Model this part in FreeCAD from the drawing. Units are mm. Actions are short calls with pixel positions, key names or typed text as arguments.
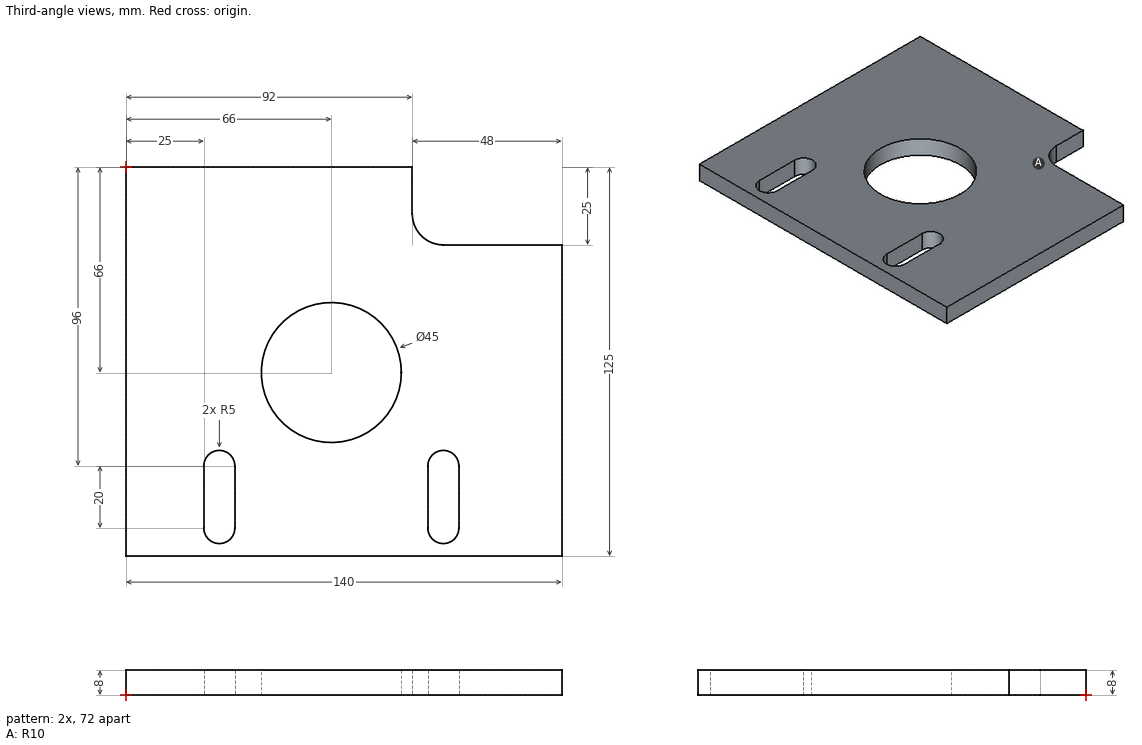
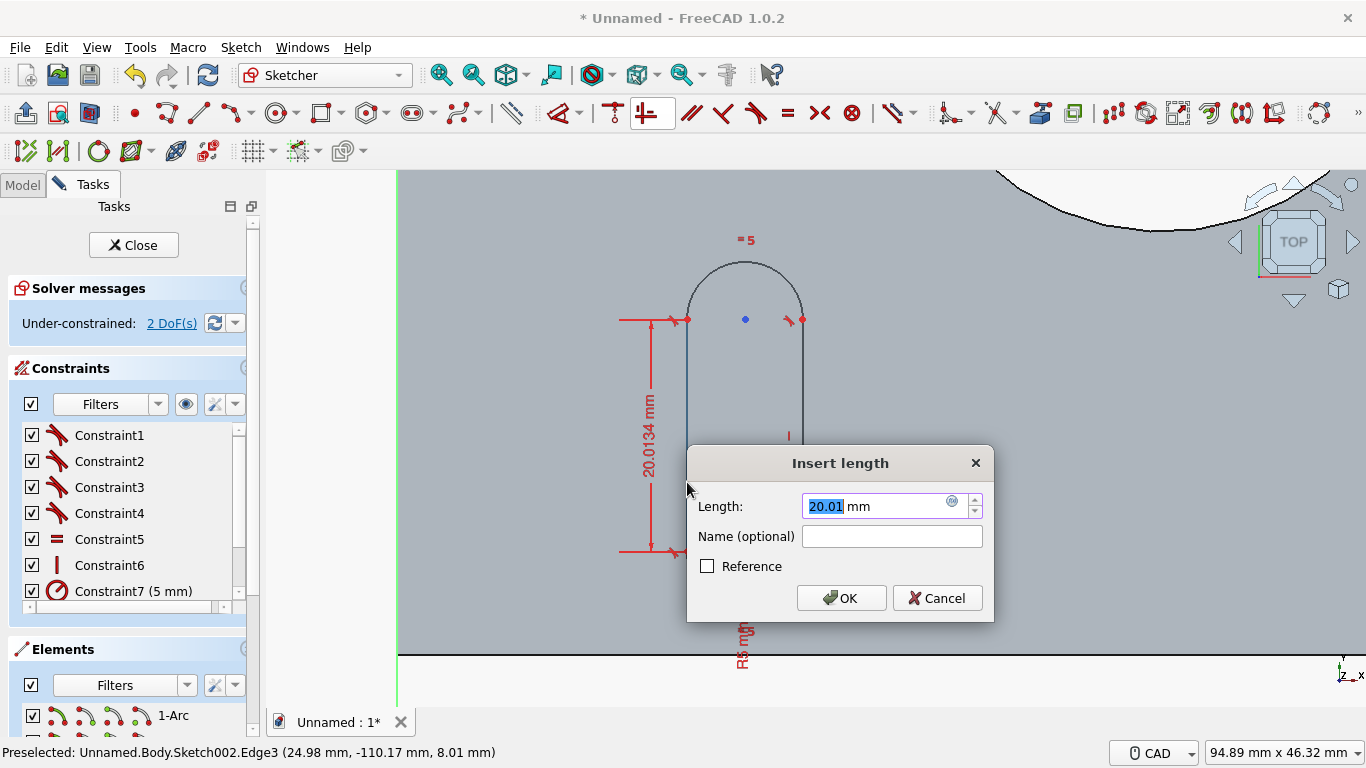
text(20)
key(Return)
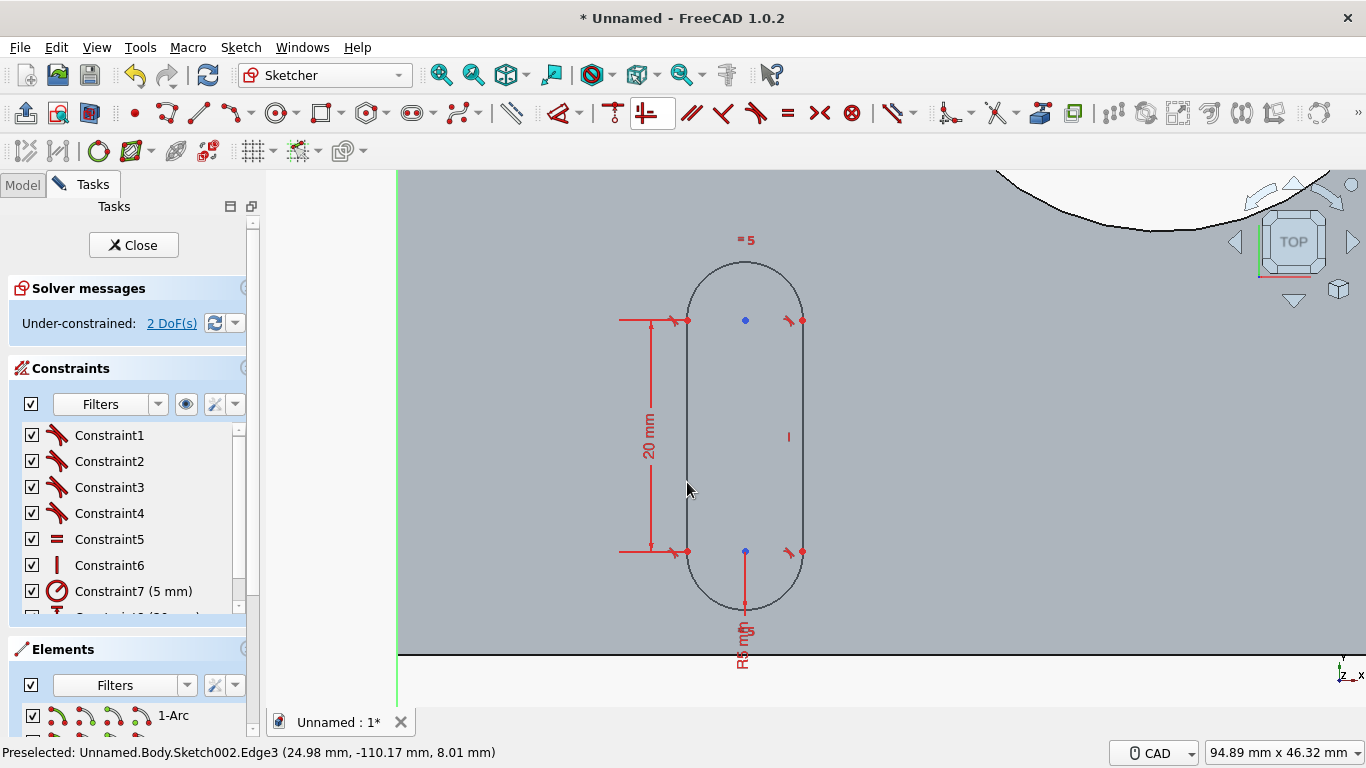
click(687, 552)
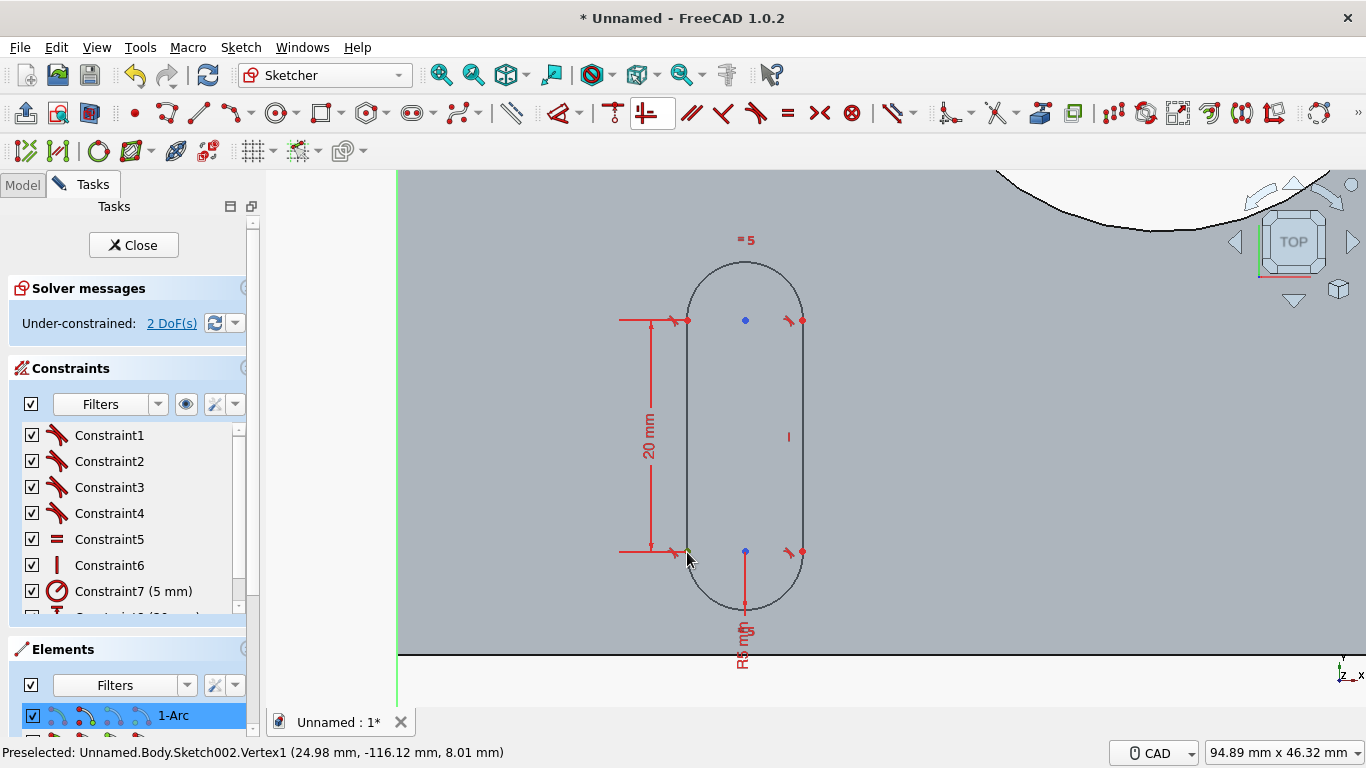
key(l)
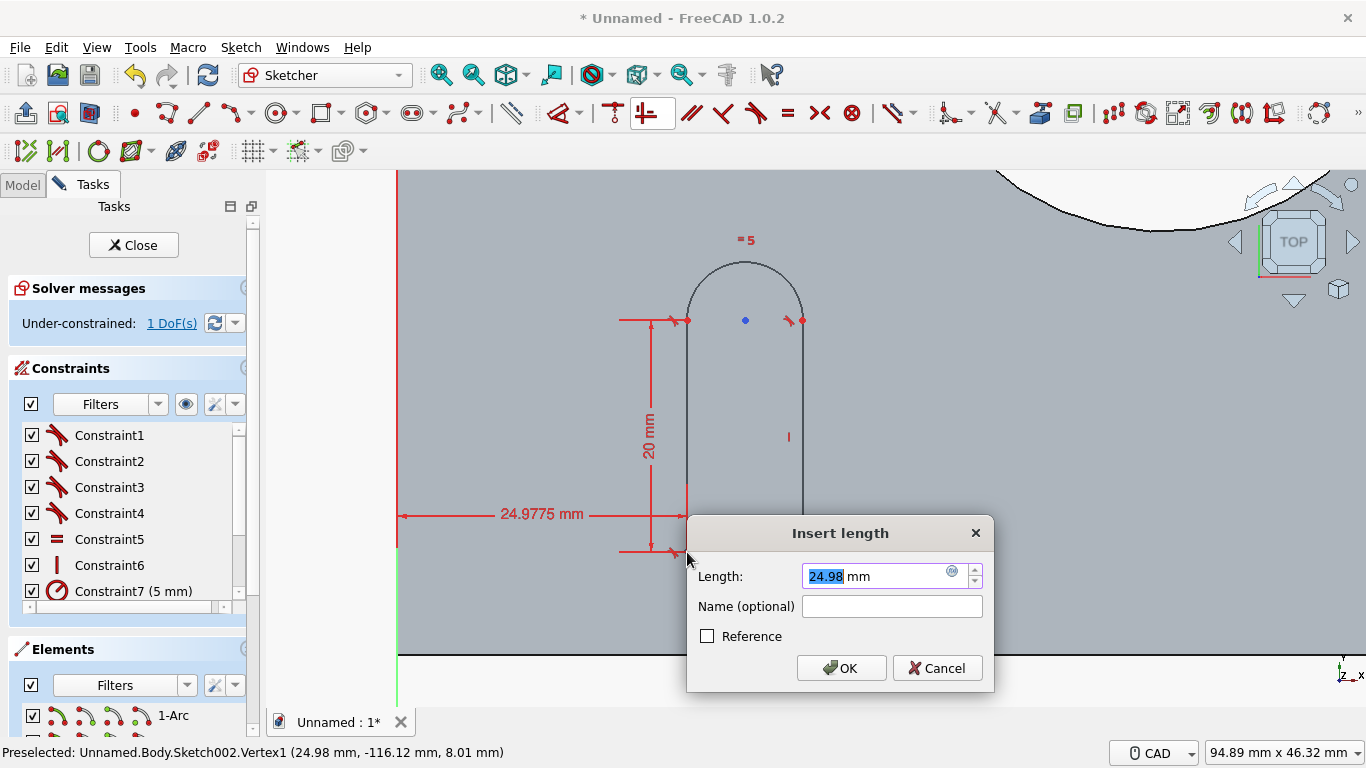
text(25)
key(Return)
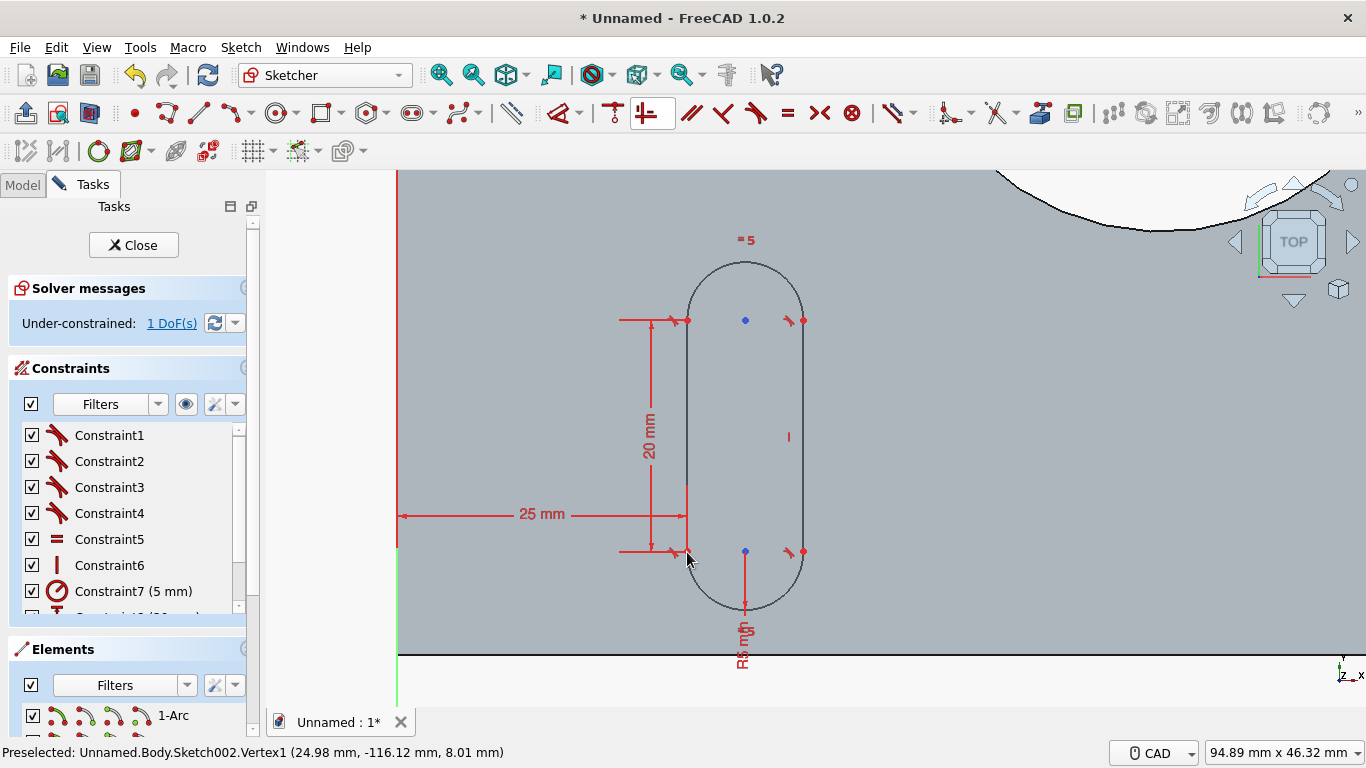
click(803, 320)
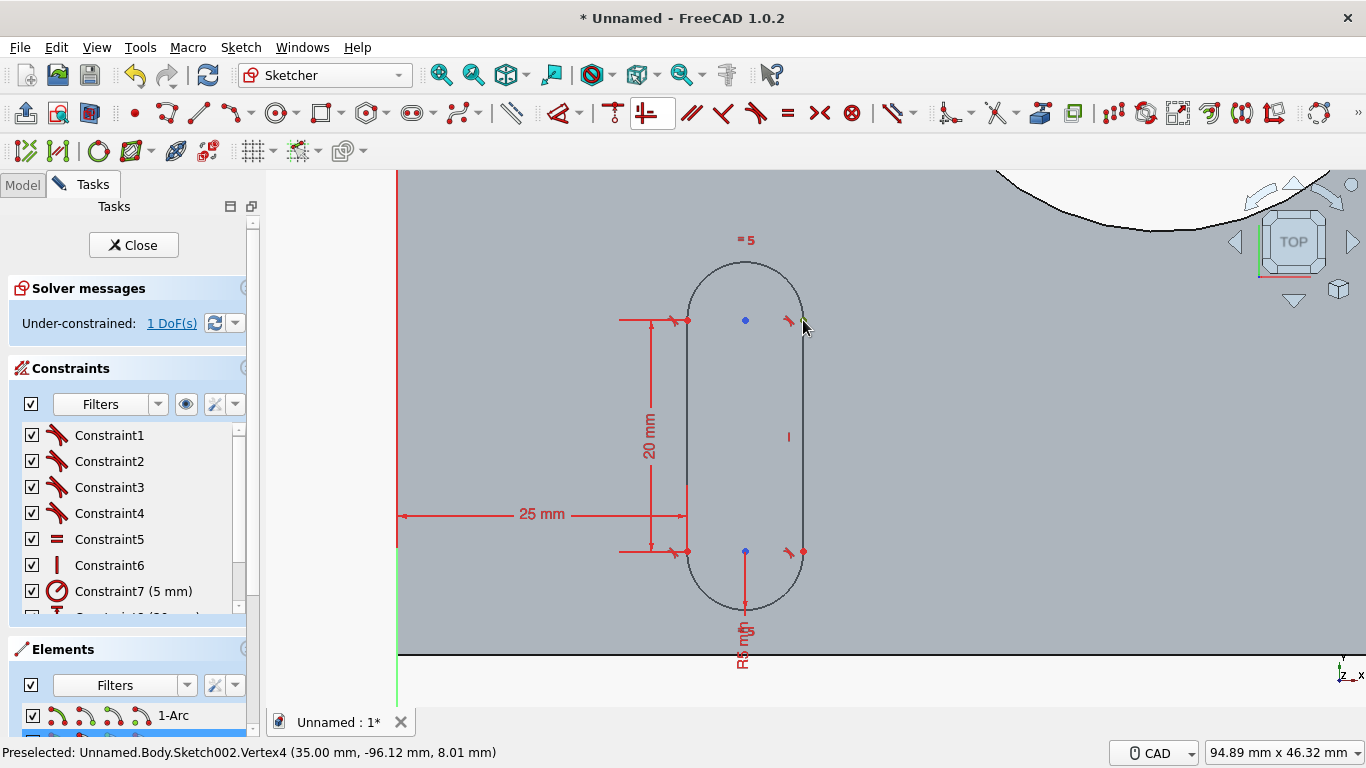
click(582, 114)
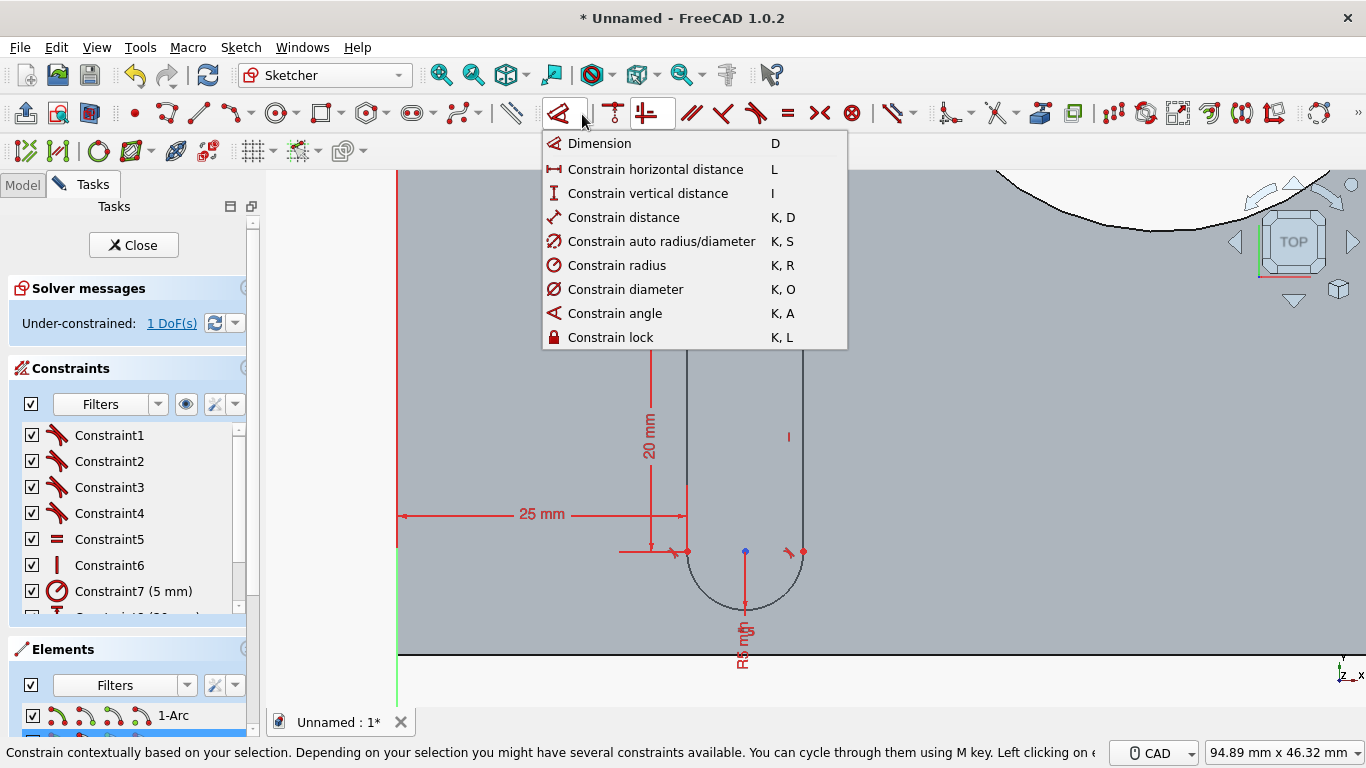
click(695, 193)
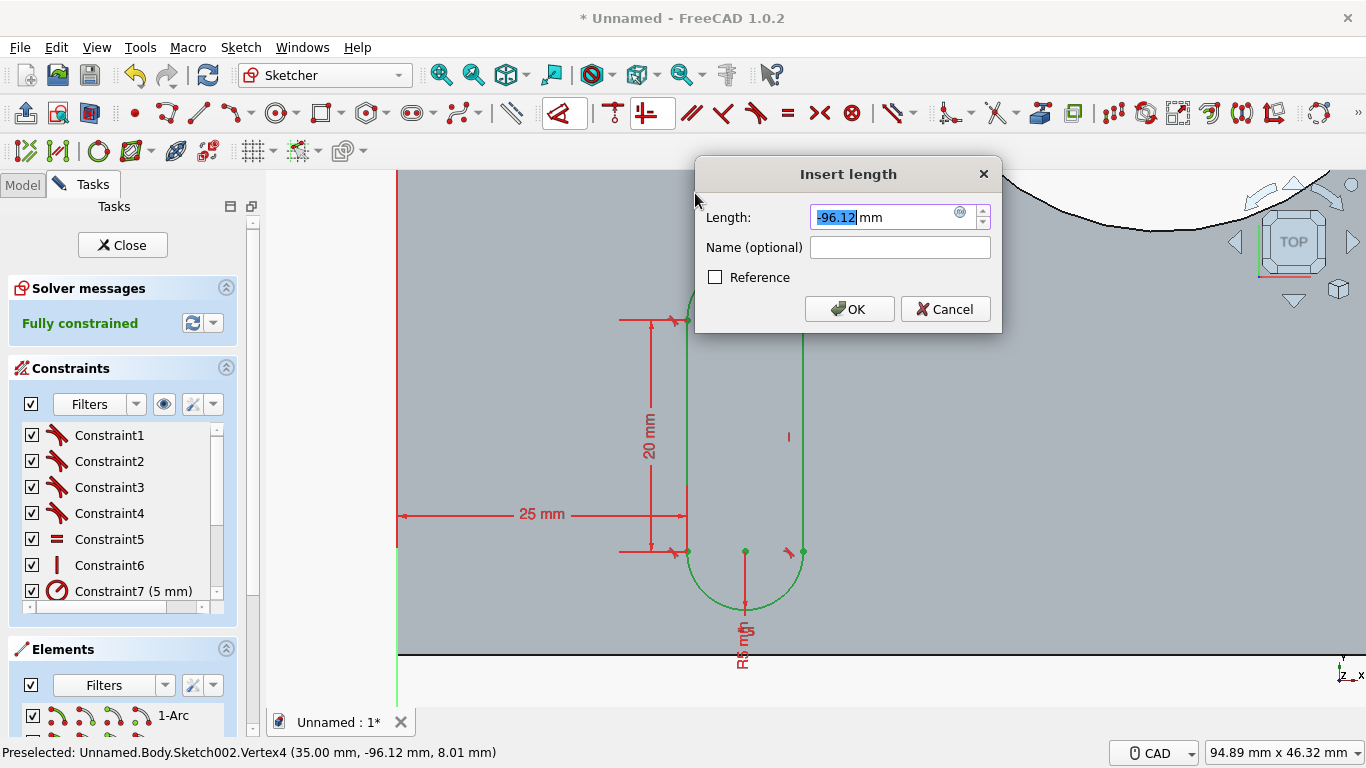
text(-96)
key(Return)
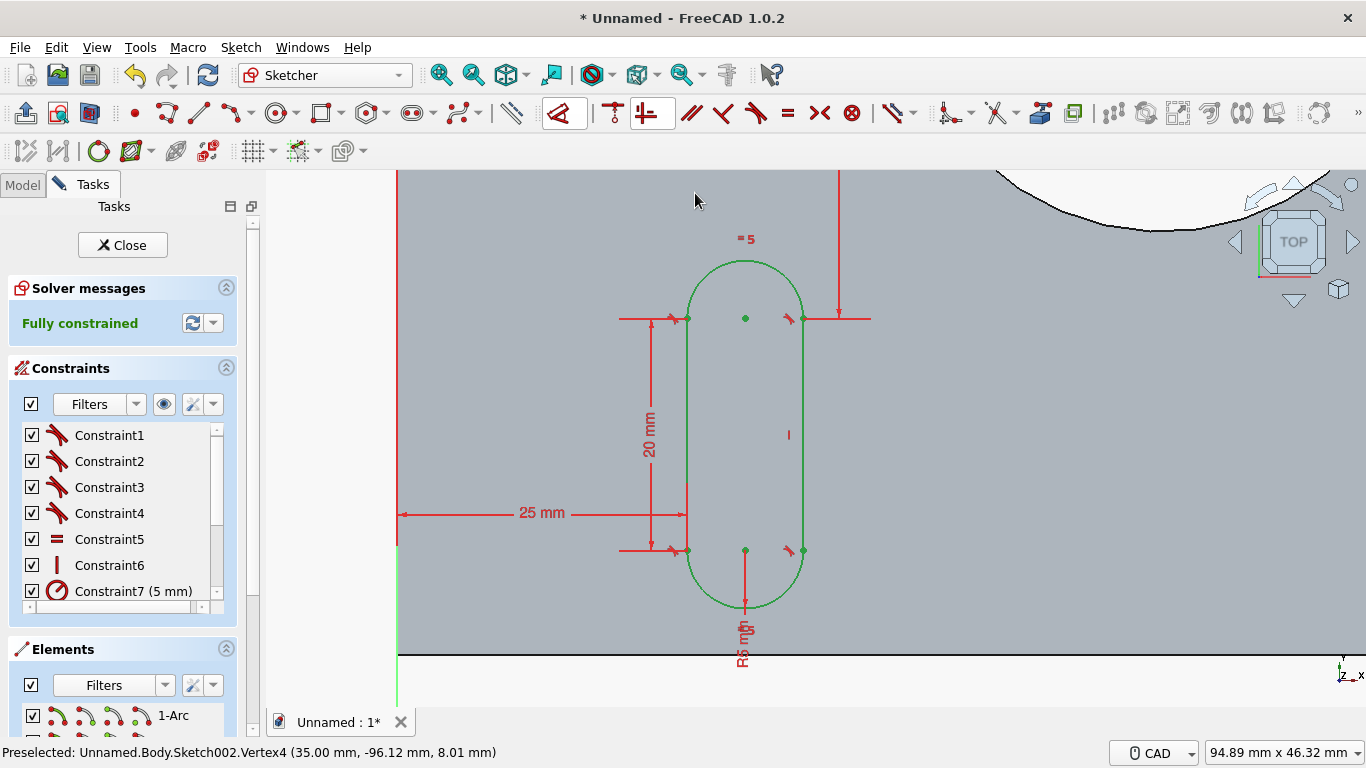
click(123, 245)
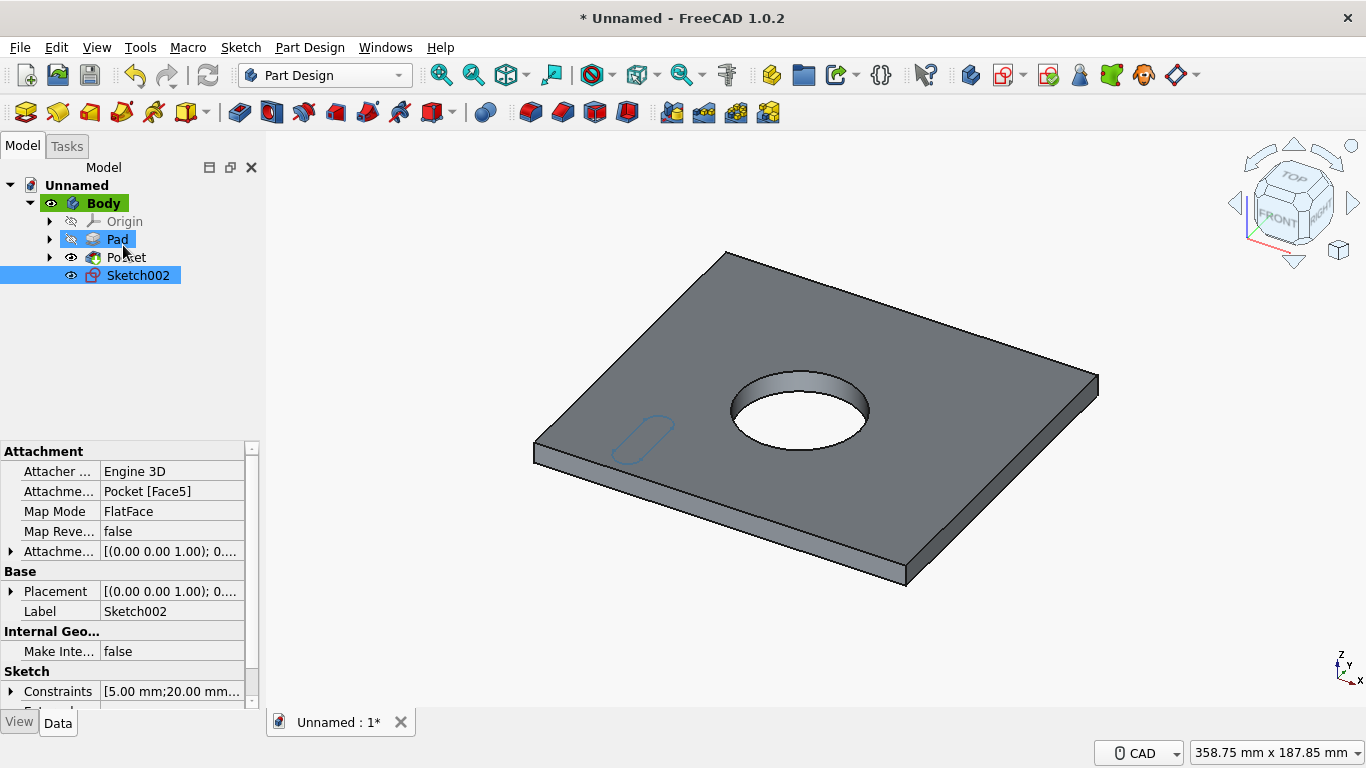
click(240, 112)